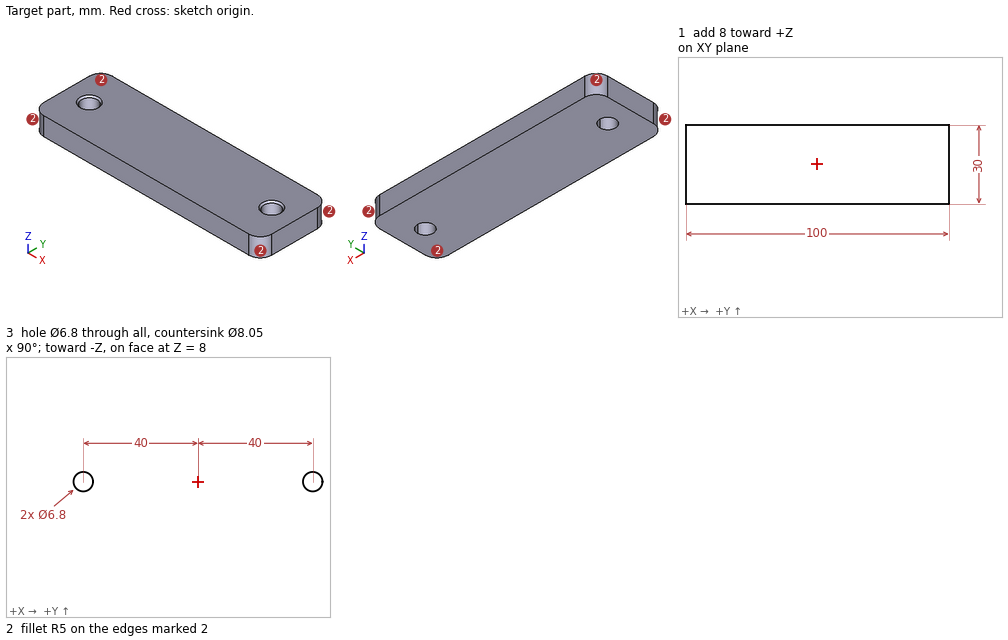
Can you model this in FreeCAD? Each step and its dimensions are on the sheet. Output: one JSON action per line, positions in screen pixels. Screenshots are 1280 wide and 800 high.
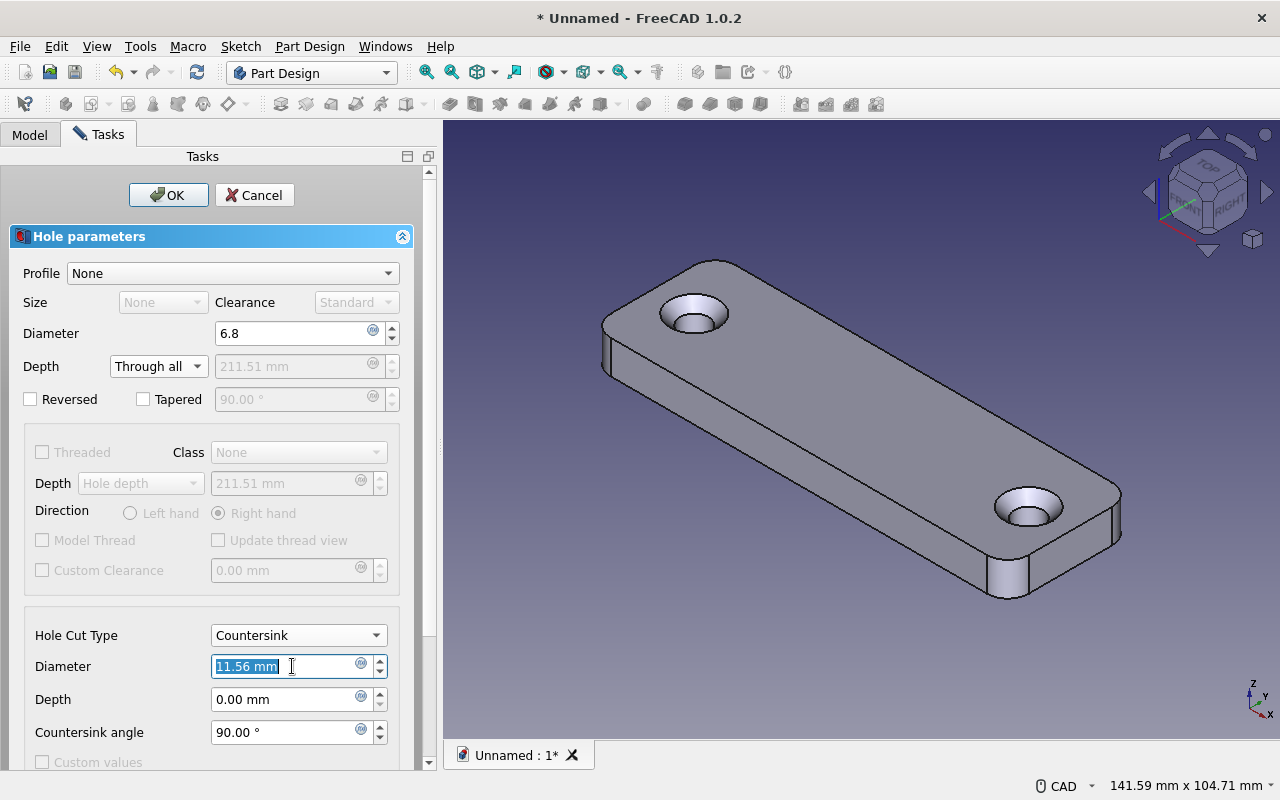
{"action": "type", "text": "8.05"}
{"action": "key", "text": "Tab"}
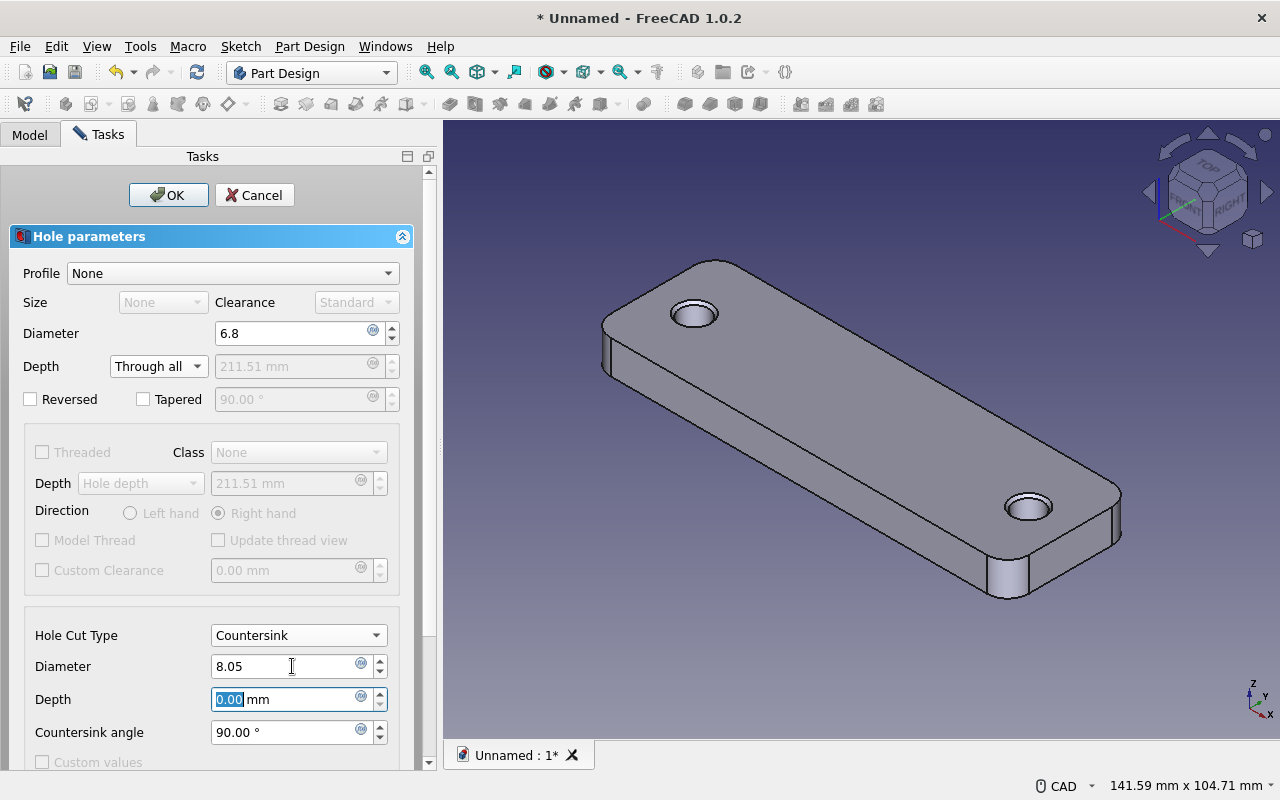
{"action": "left_click", "coordinate": [169, 195]}